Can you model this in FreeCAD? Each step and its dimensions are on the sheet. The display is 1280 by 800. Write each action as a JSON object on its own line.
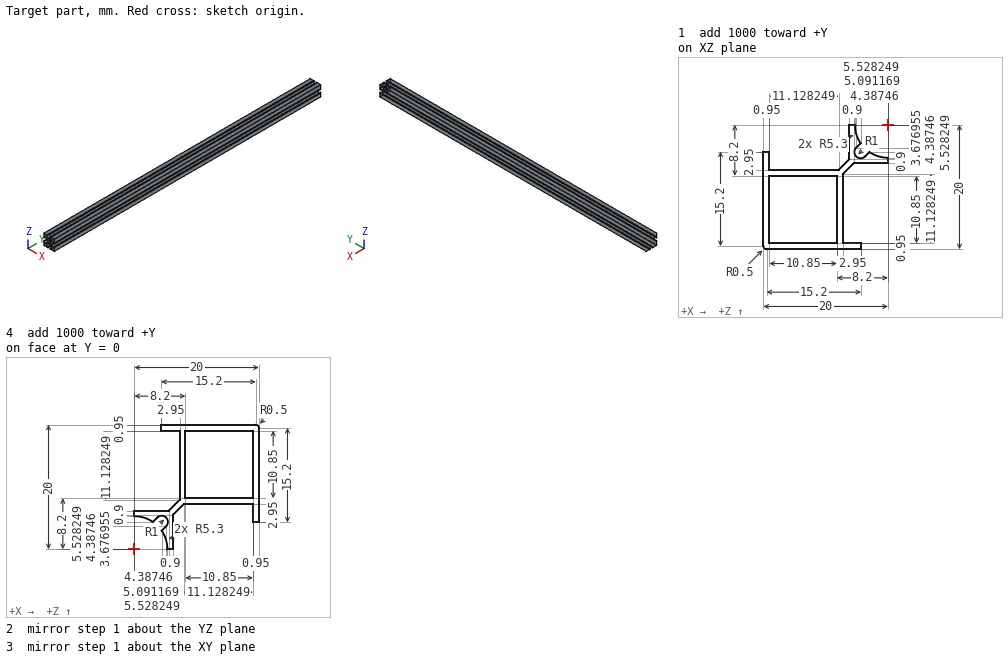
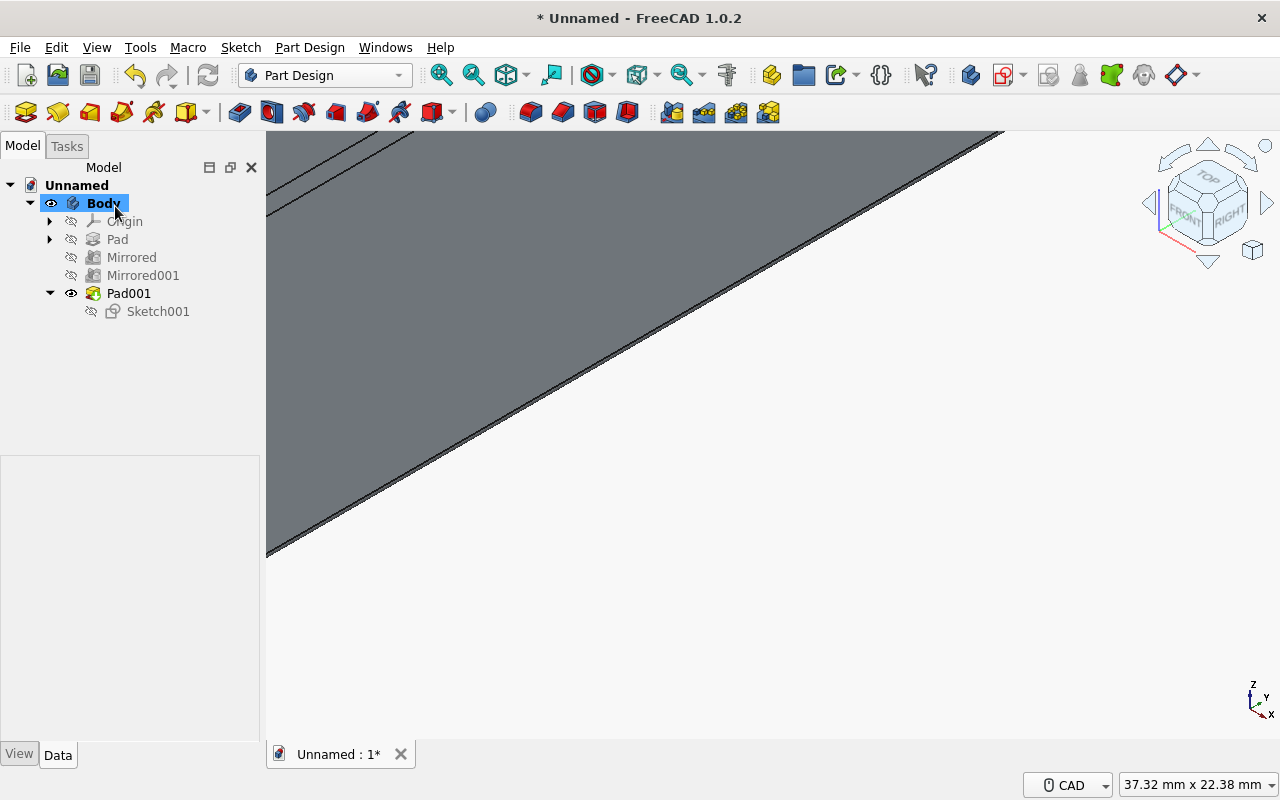
{"action": "left_click", "coordinate": [442, 76]}